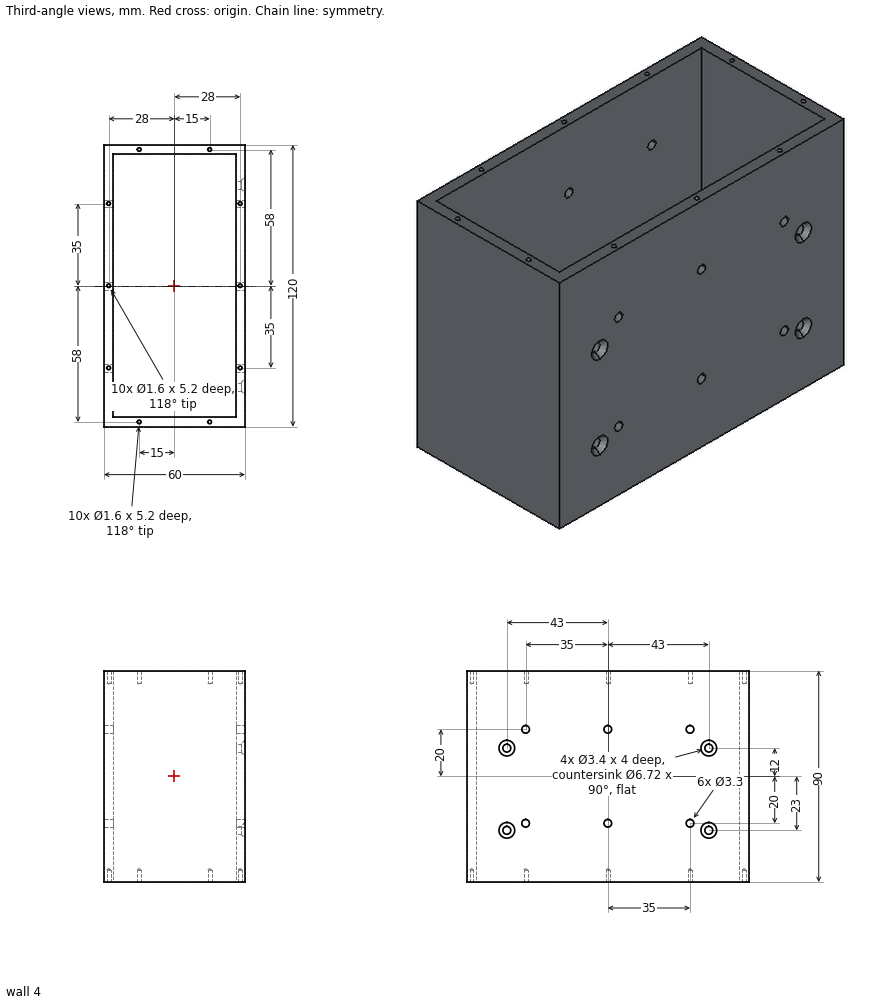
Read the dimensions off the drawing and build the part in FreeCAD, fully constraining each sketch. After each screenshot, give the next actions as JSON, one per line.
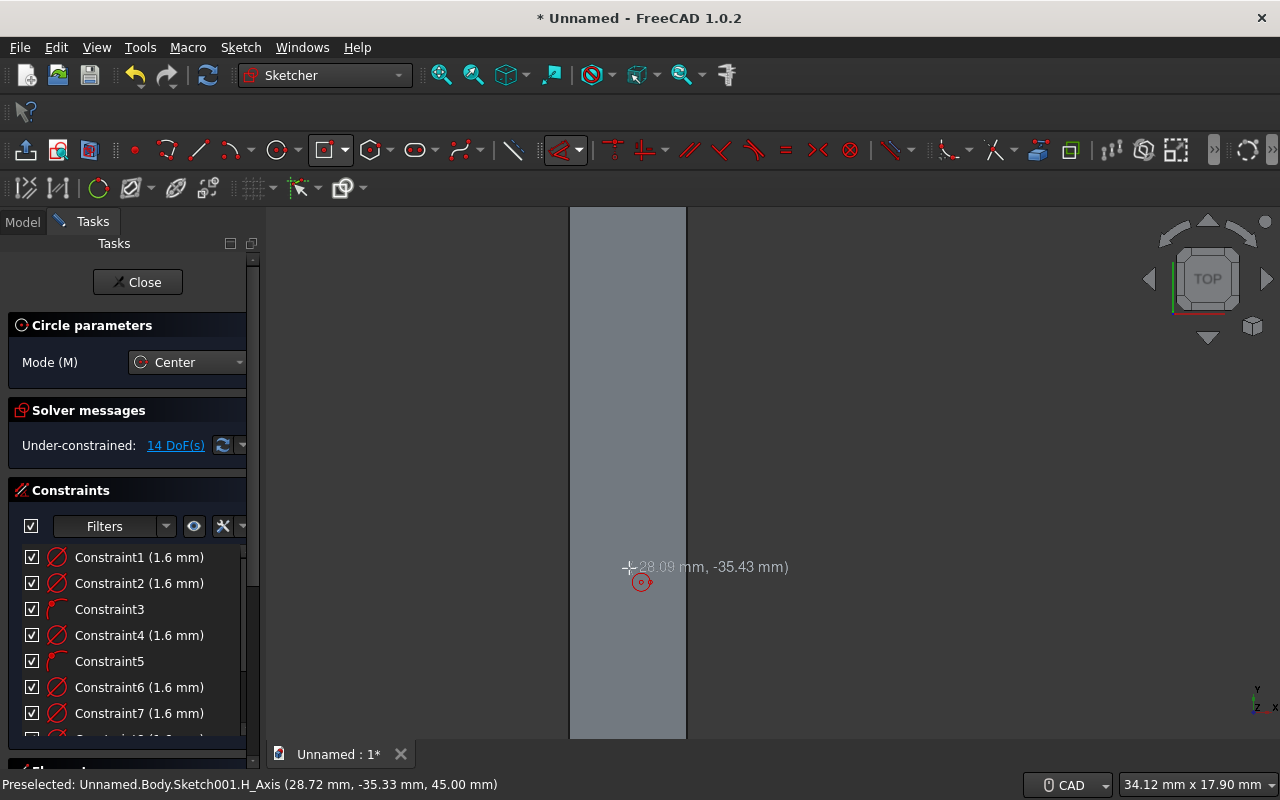
{"action": "scroll", "coordinate": [629, 568], "scroll_direction": "down", "scroll_amount": 12}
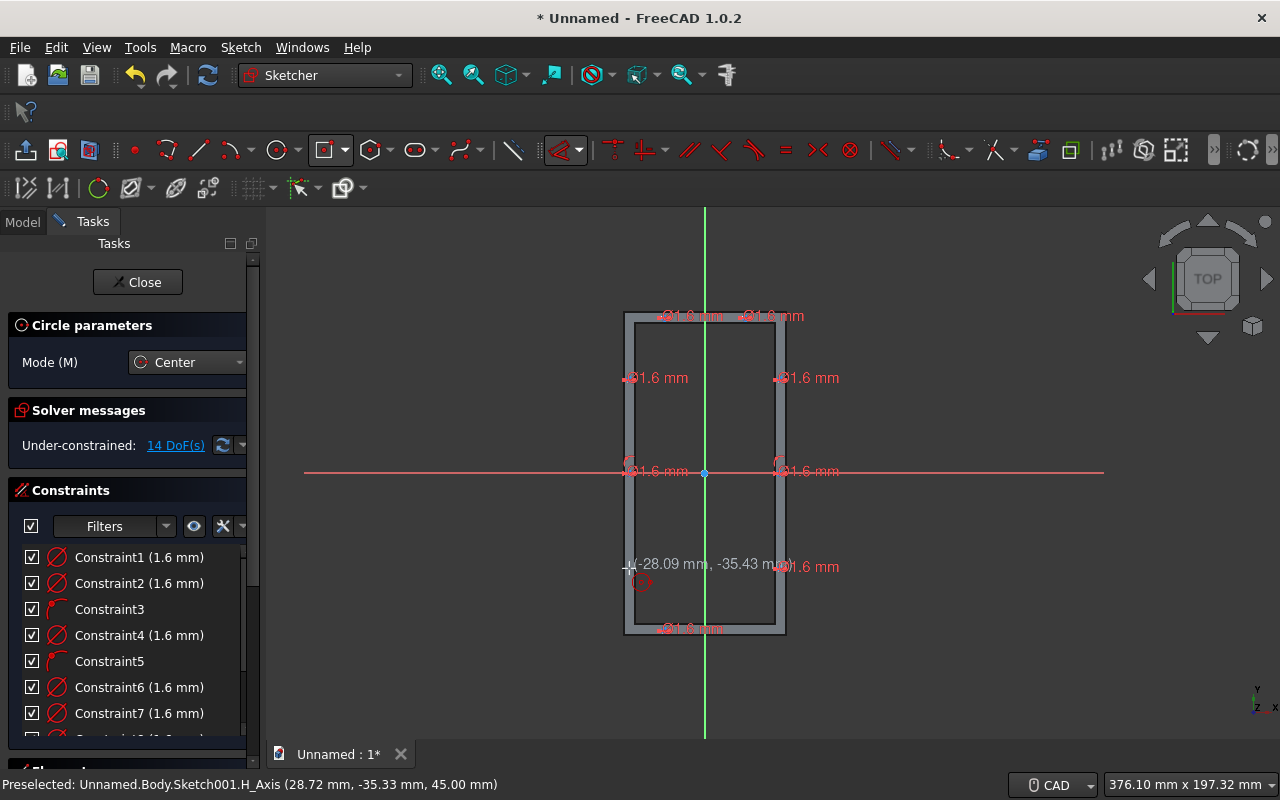
{"action": "left_click", "coordinate": [629, 568]}
{"action": "mouse_move", "coordinate": [631, 566]}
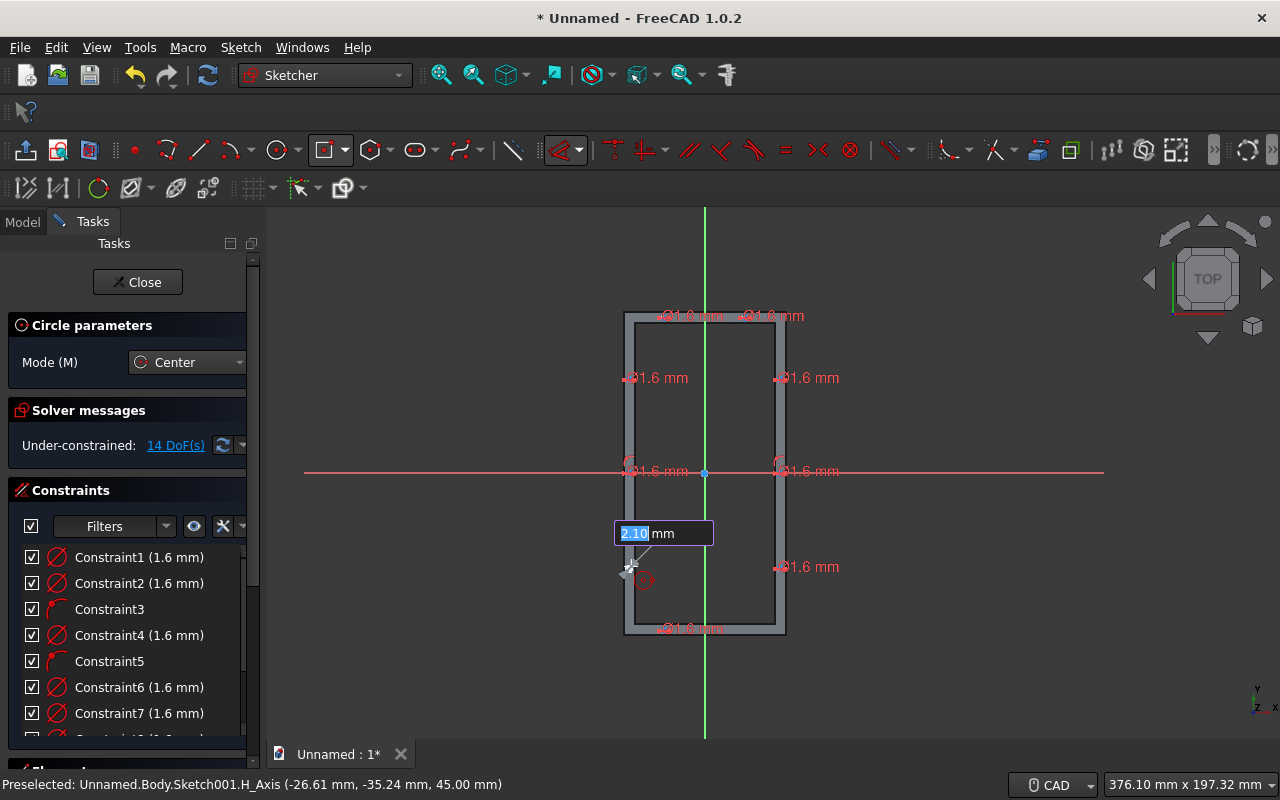
{"action": "type", "text": "1.6"}
{"action": "key", "text": "Return"}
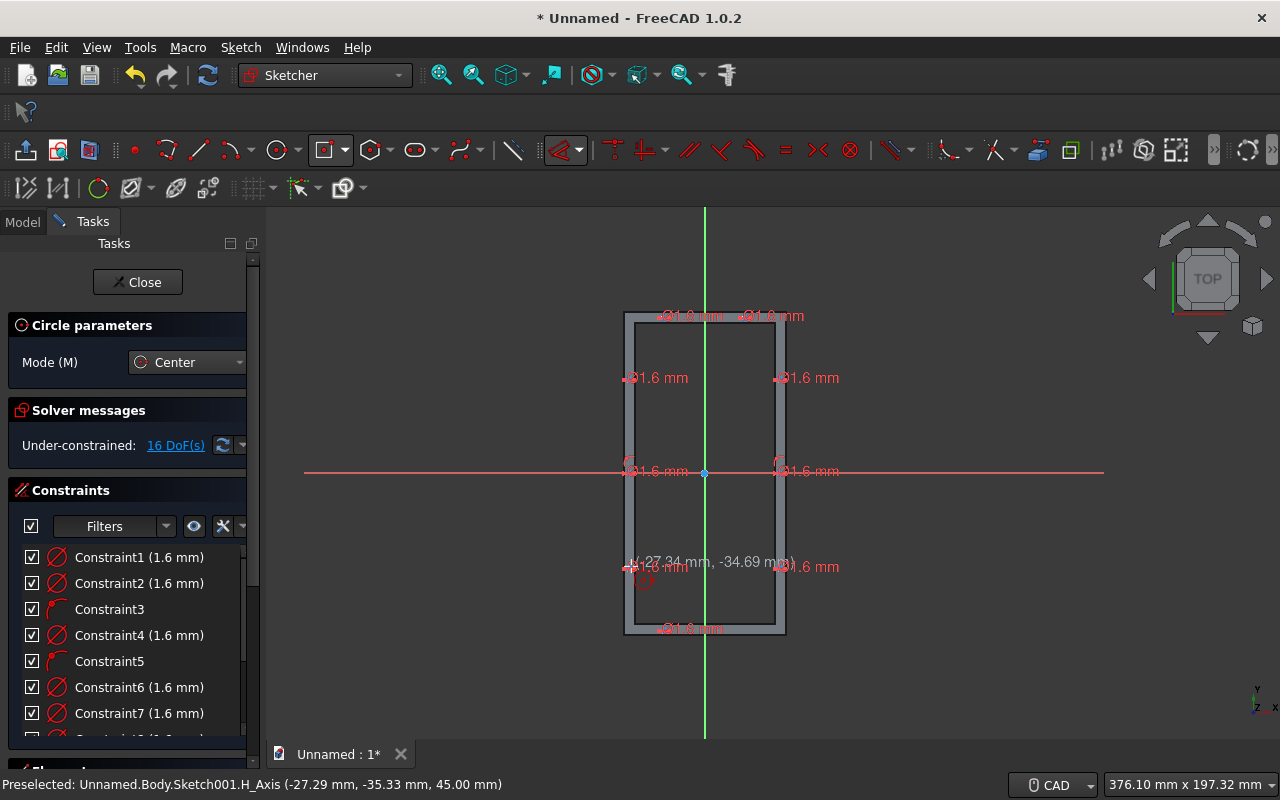
{"action": "scroll", "coordinate": [745, 630], "scroll_direction": "up", "scroll_amount": 12}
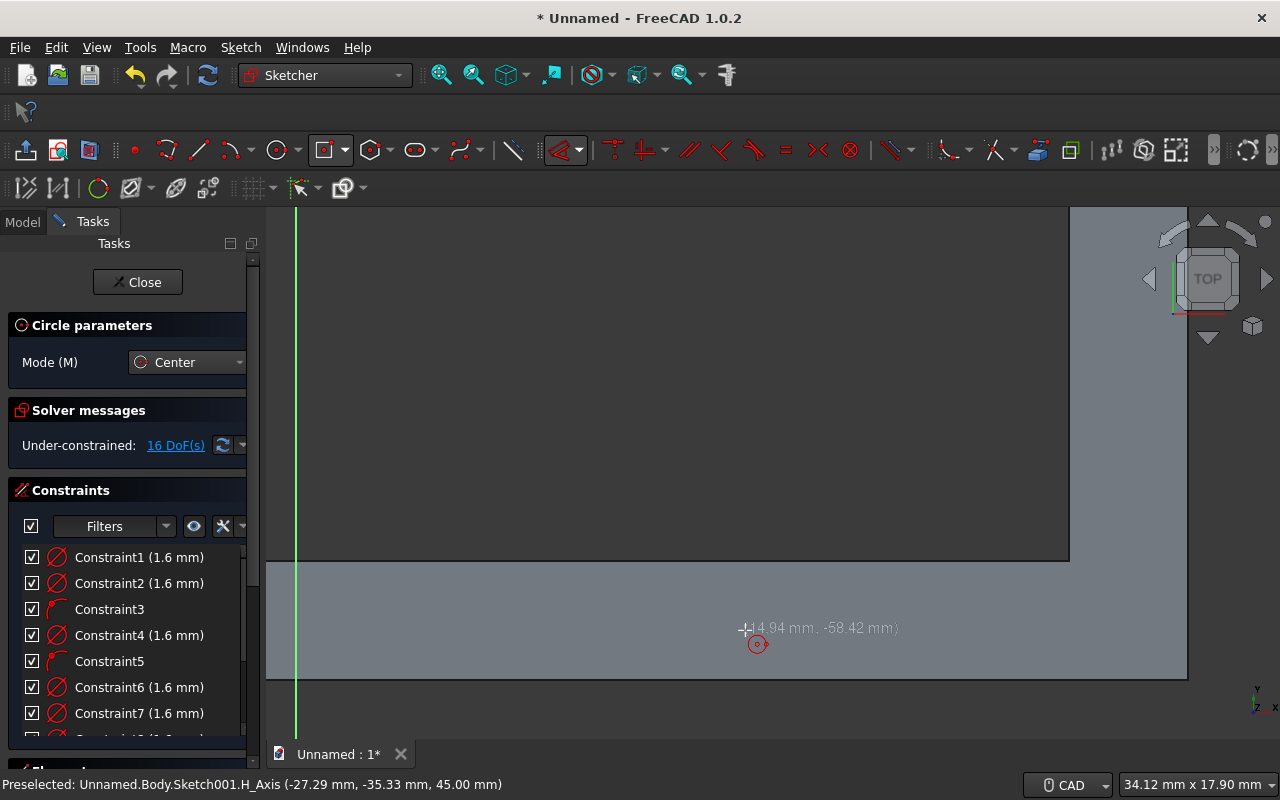
{"action": "scroll", "coordinate": [745, 630], "scroll_direction": "down", "scroll_amount": 12}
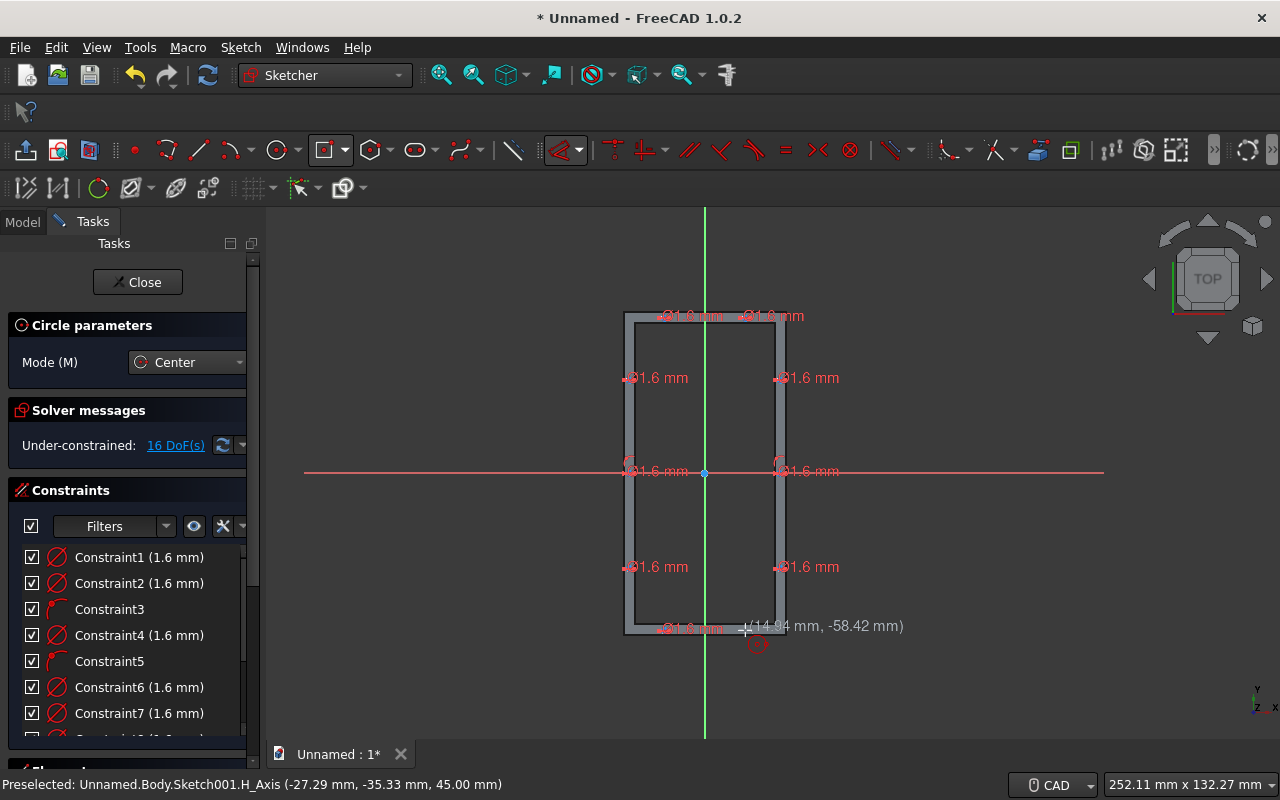
{"action": "left_click", "coordinate": [745, 630]}
{"action": "mouse_move", "coordinate": [747, 628]}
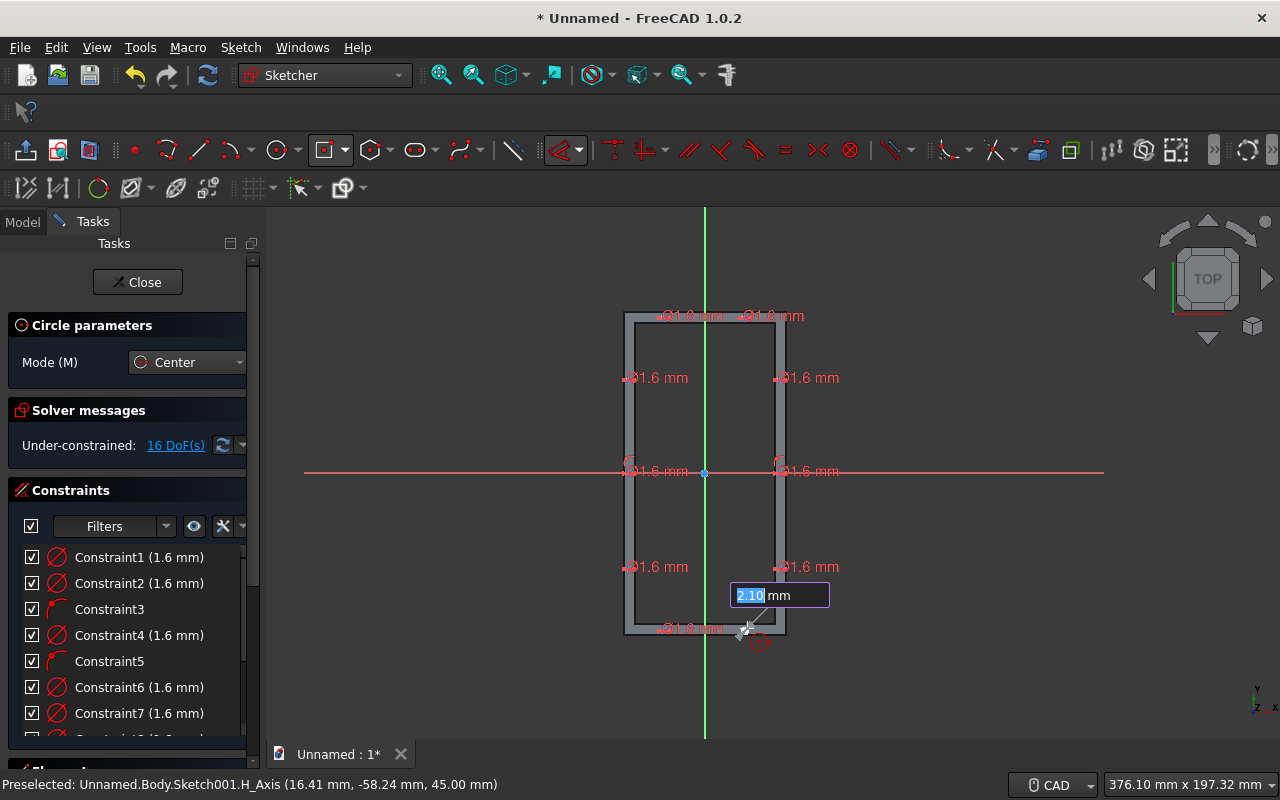
{"action": "type", "text": "1.6"}
{"action": "key", "text": "Return"}
{"action": "key", "text": "Escape"}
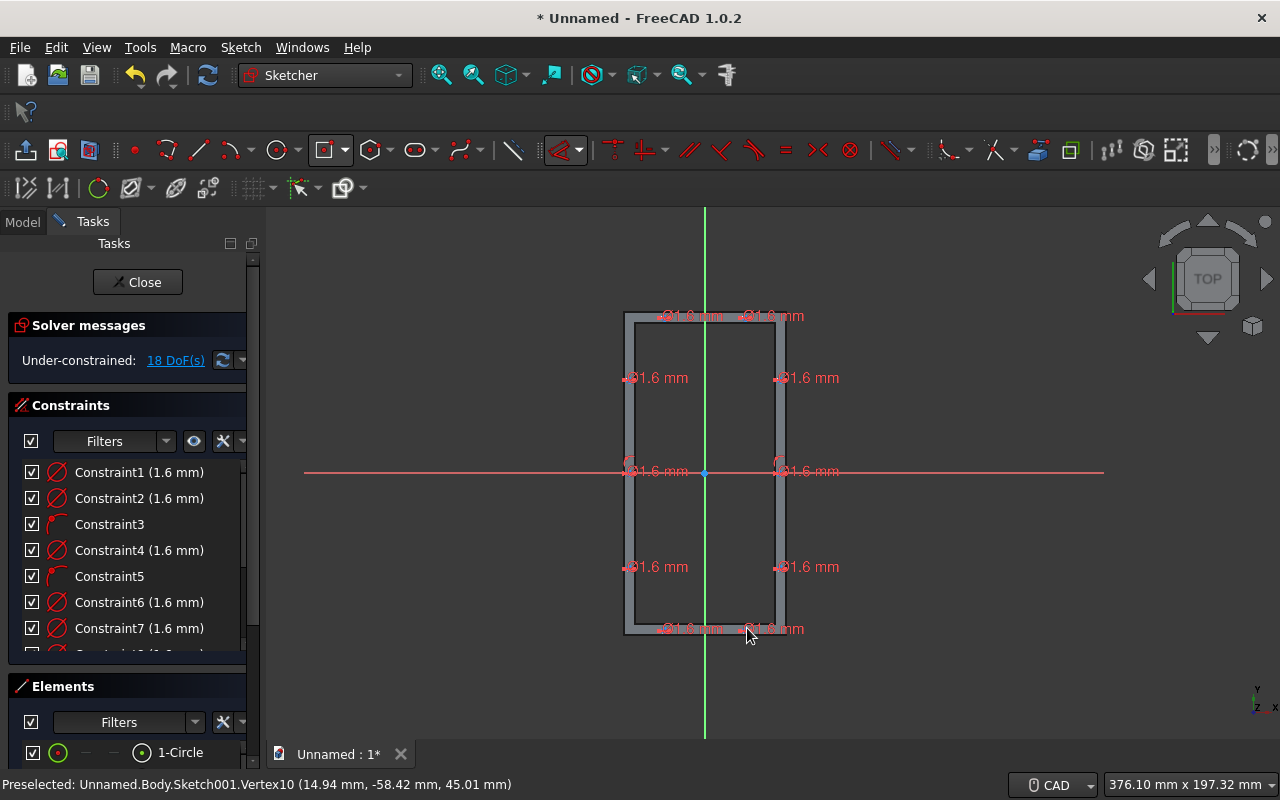
{"action": "left_click", "coordinate": [664, 631]}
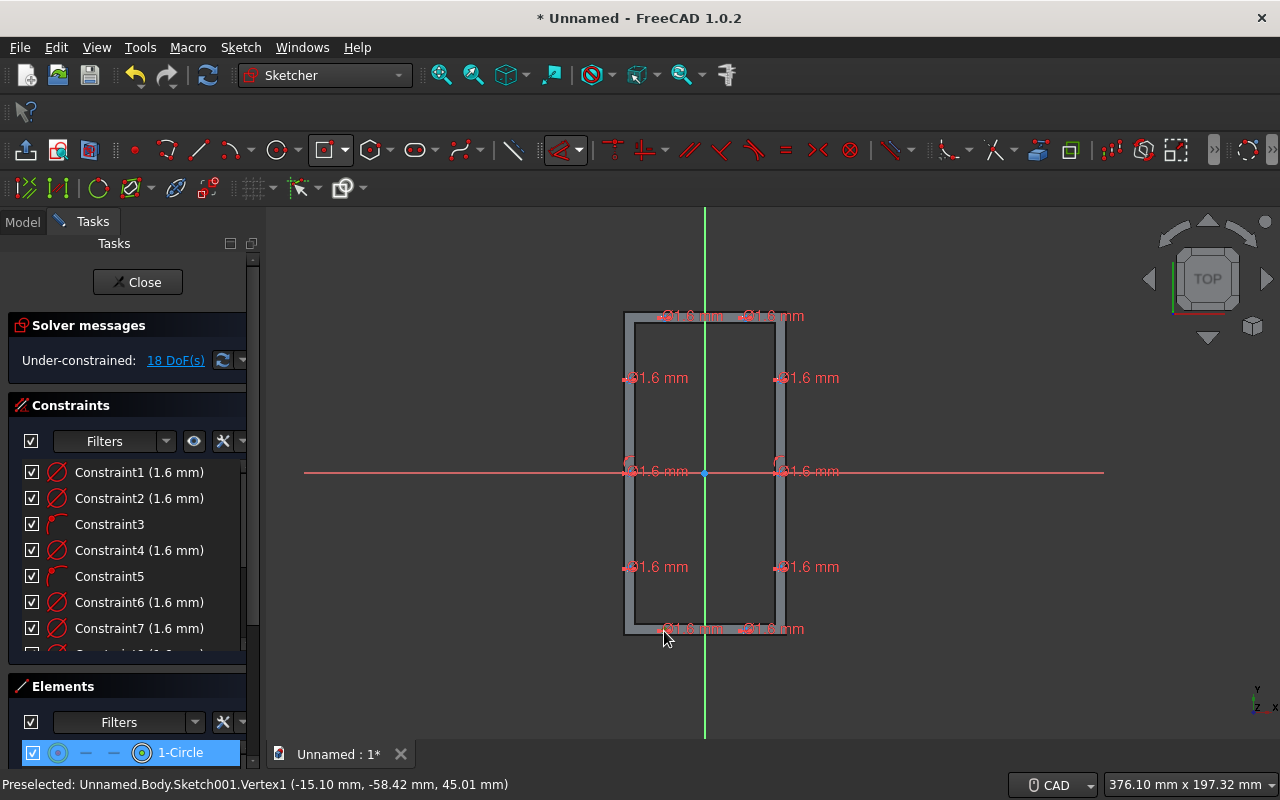
{"action": "left_click", "coordinate": [664, 318]}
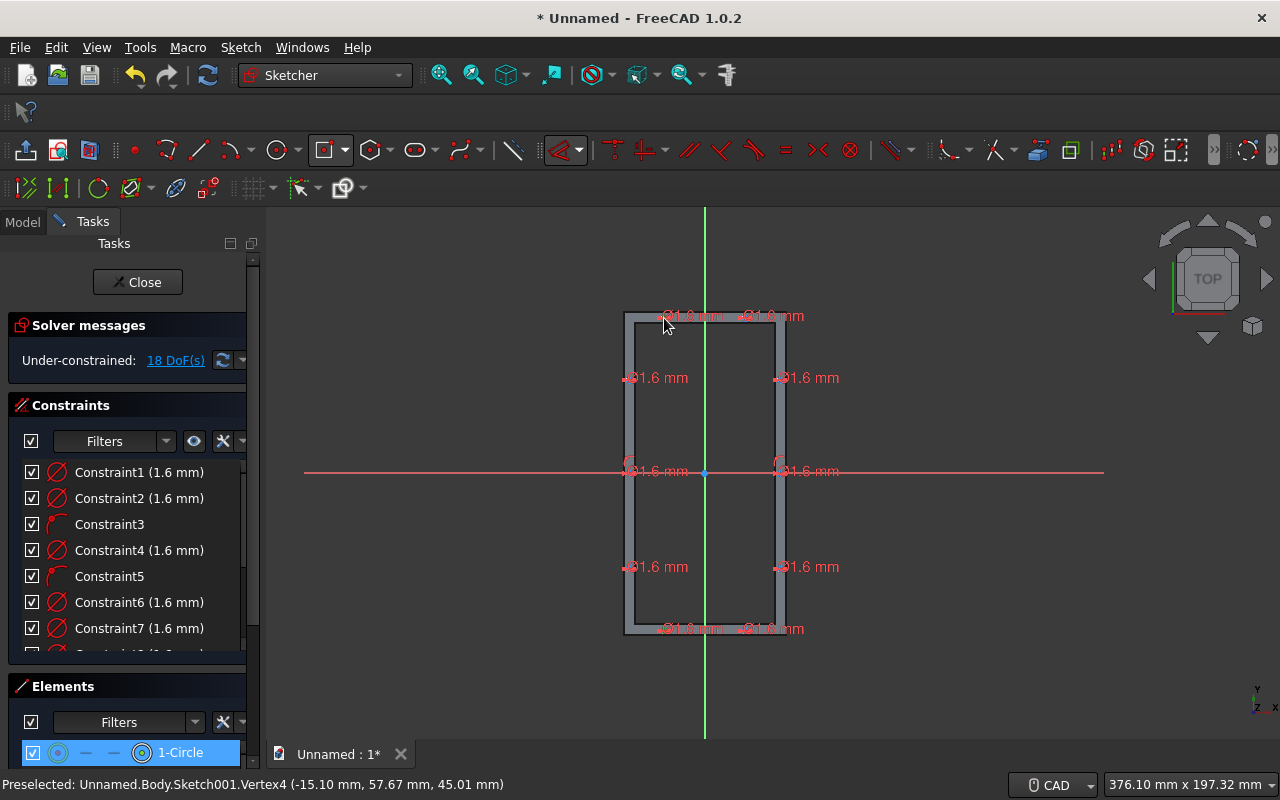
{"action": "key", "text": "v"}